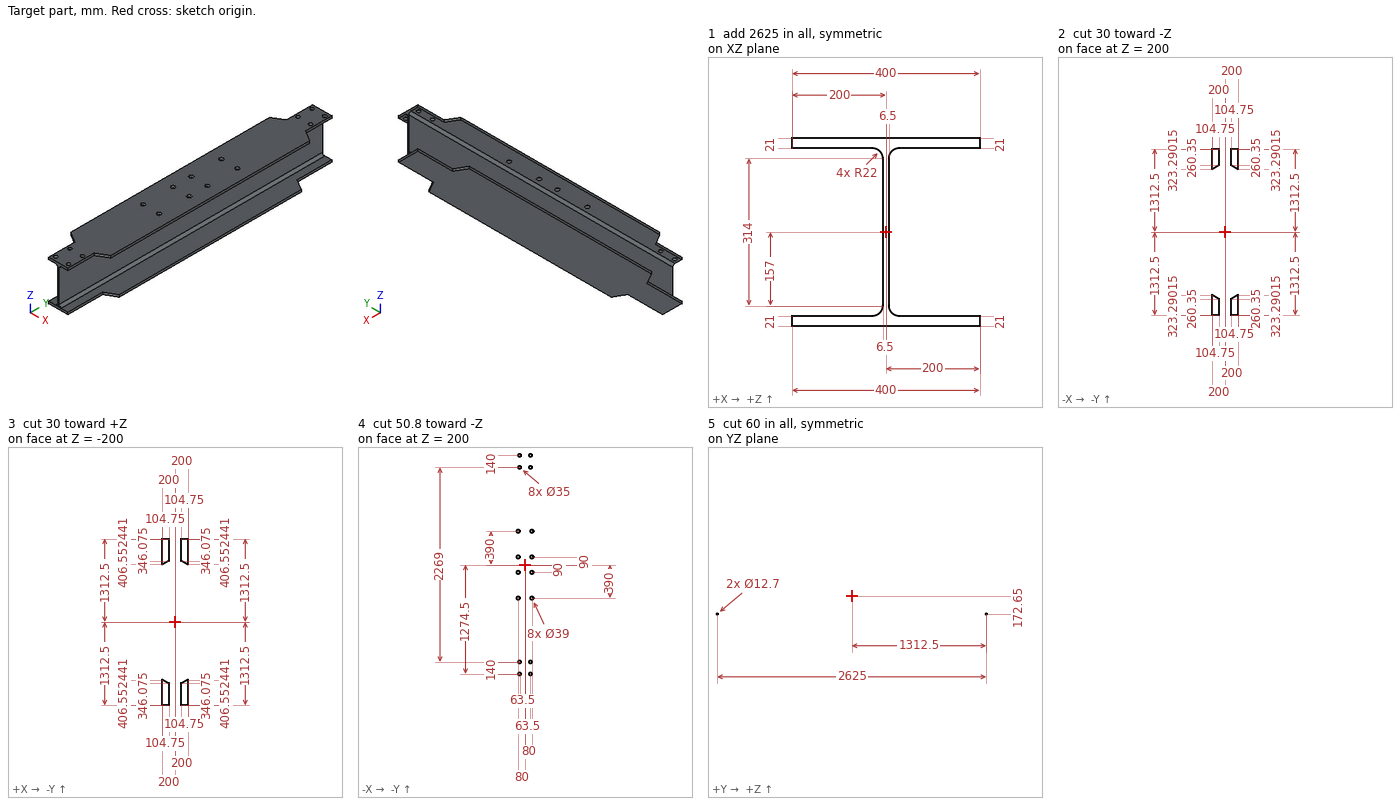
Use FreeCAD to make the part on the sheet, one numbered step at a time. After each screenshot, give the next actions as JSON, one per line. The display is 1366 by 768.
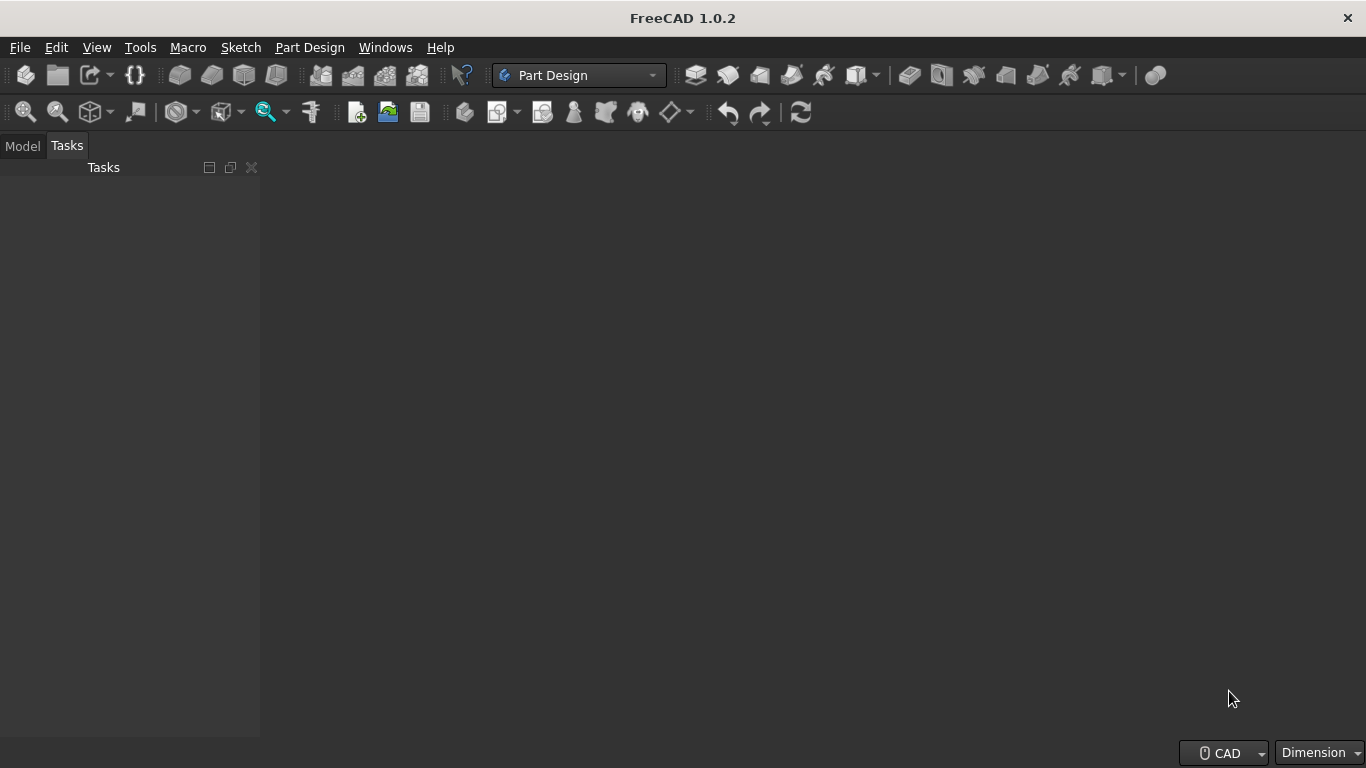
{"action": "left_click", "coordinate": [356, 112]}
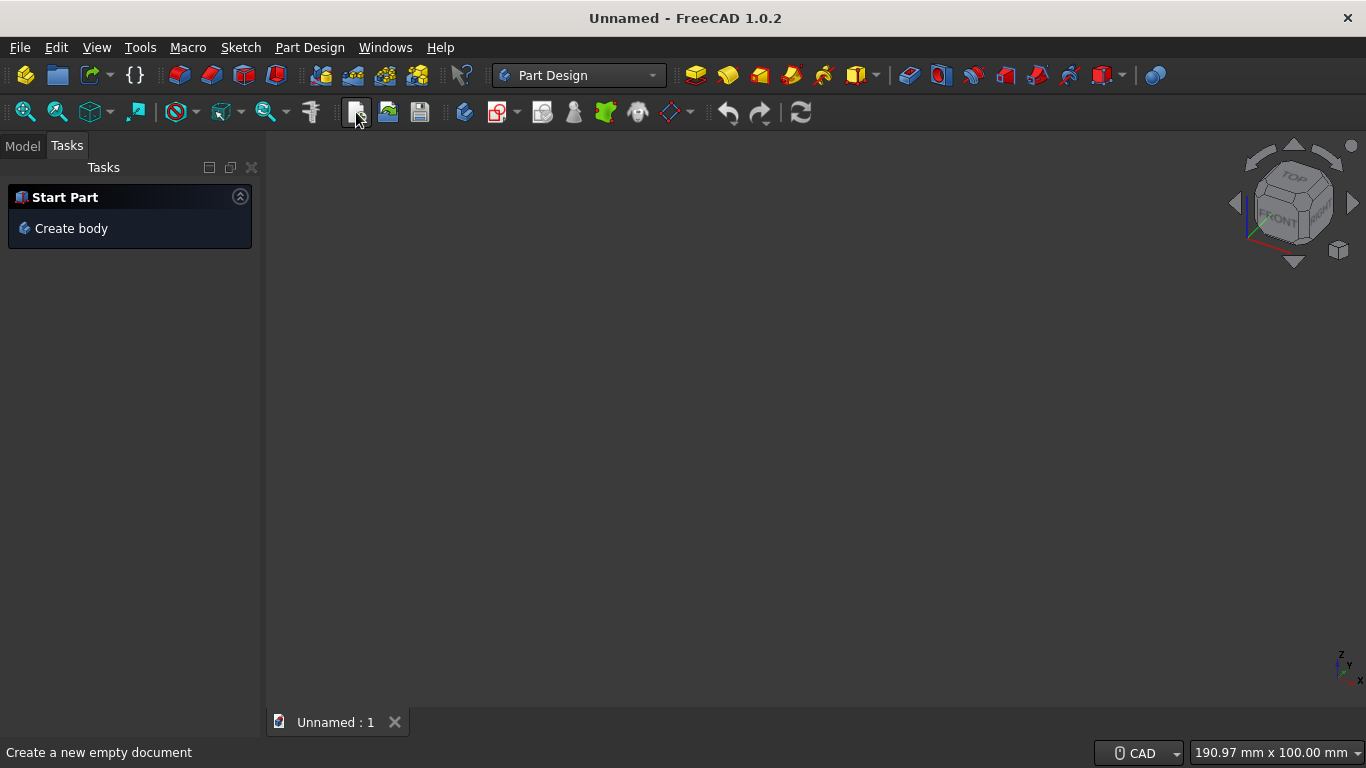
{"action": "left_click", "coordinate": [498, 112]}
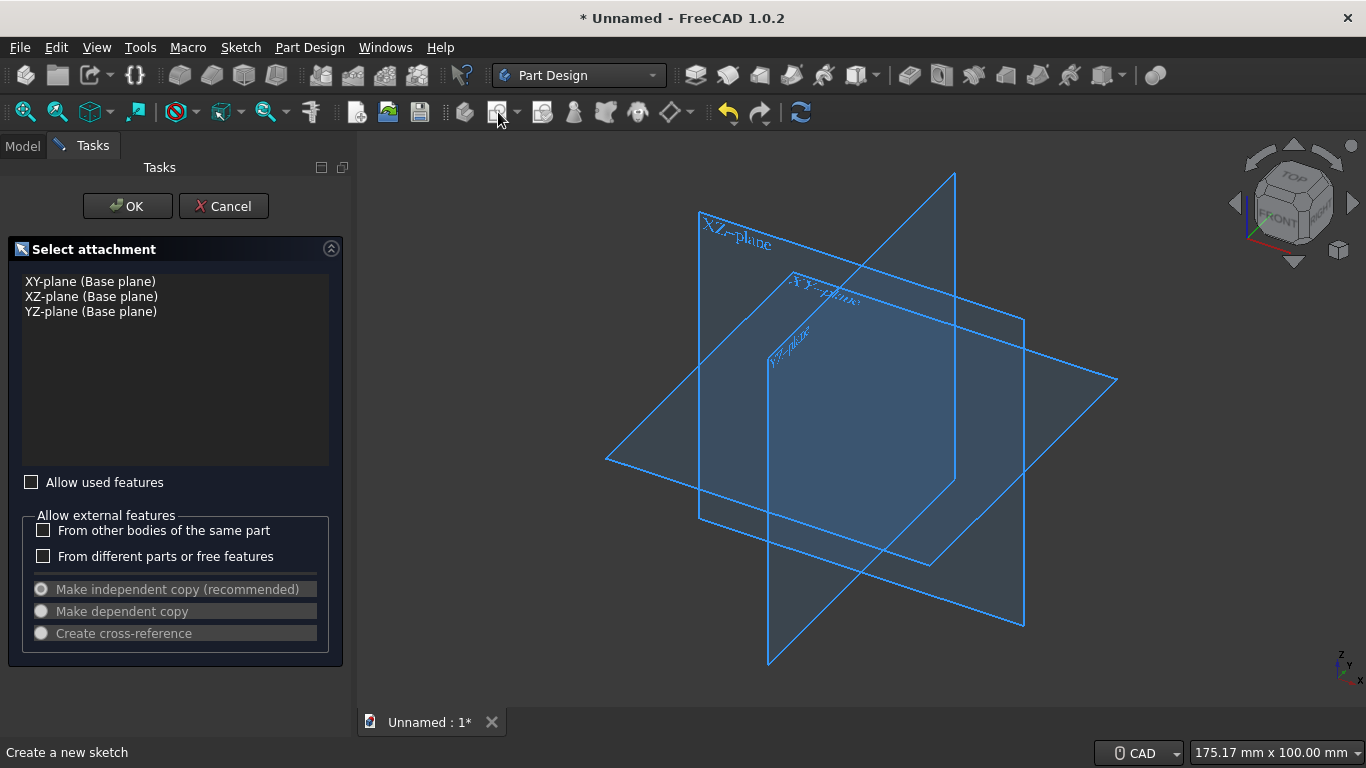
{"action": "left_click", "coordinate": [82, 296]}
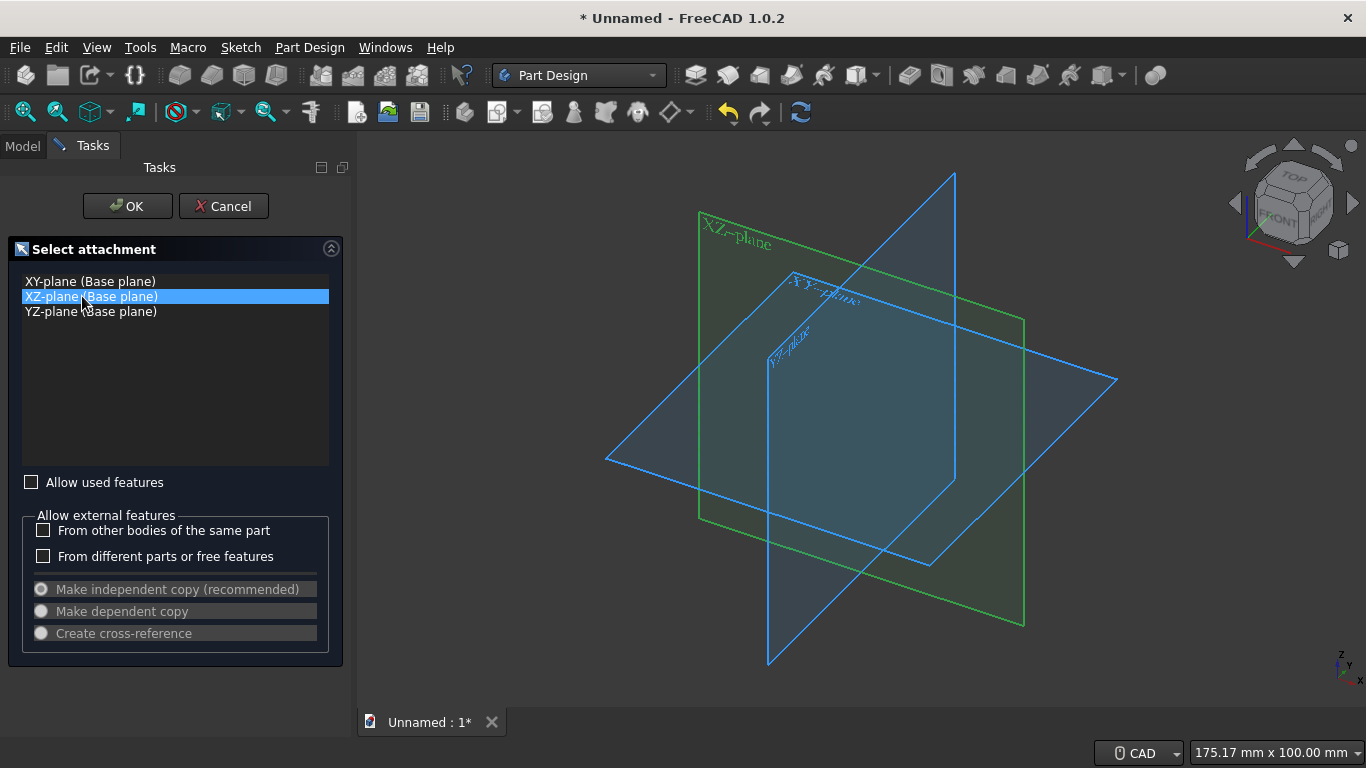
{"action": "left_click", "coordinate": [128, 206]}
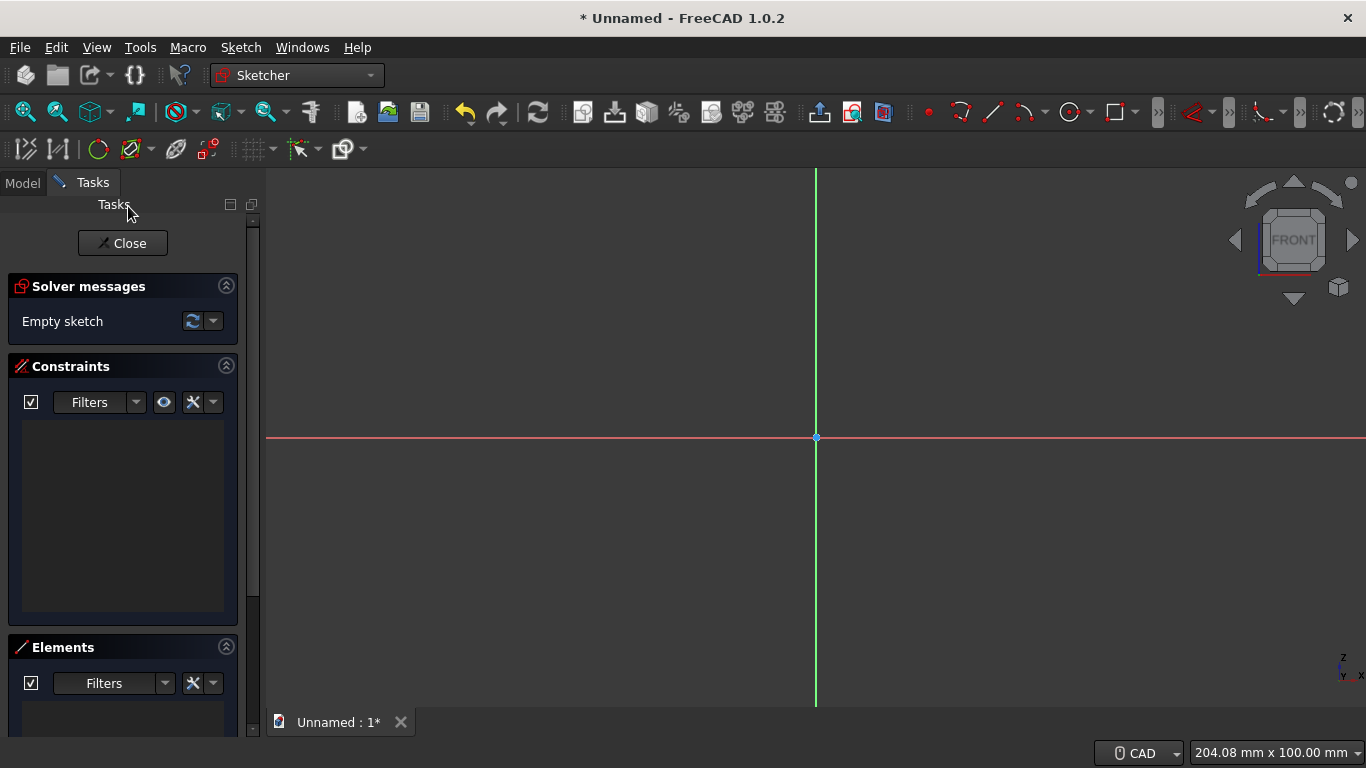
{"action": "scroll", "coordinate": [734, 438], "scroll_direction": "down", "scroll_amount": 9}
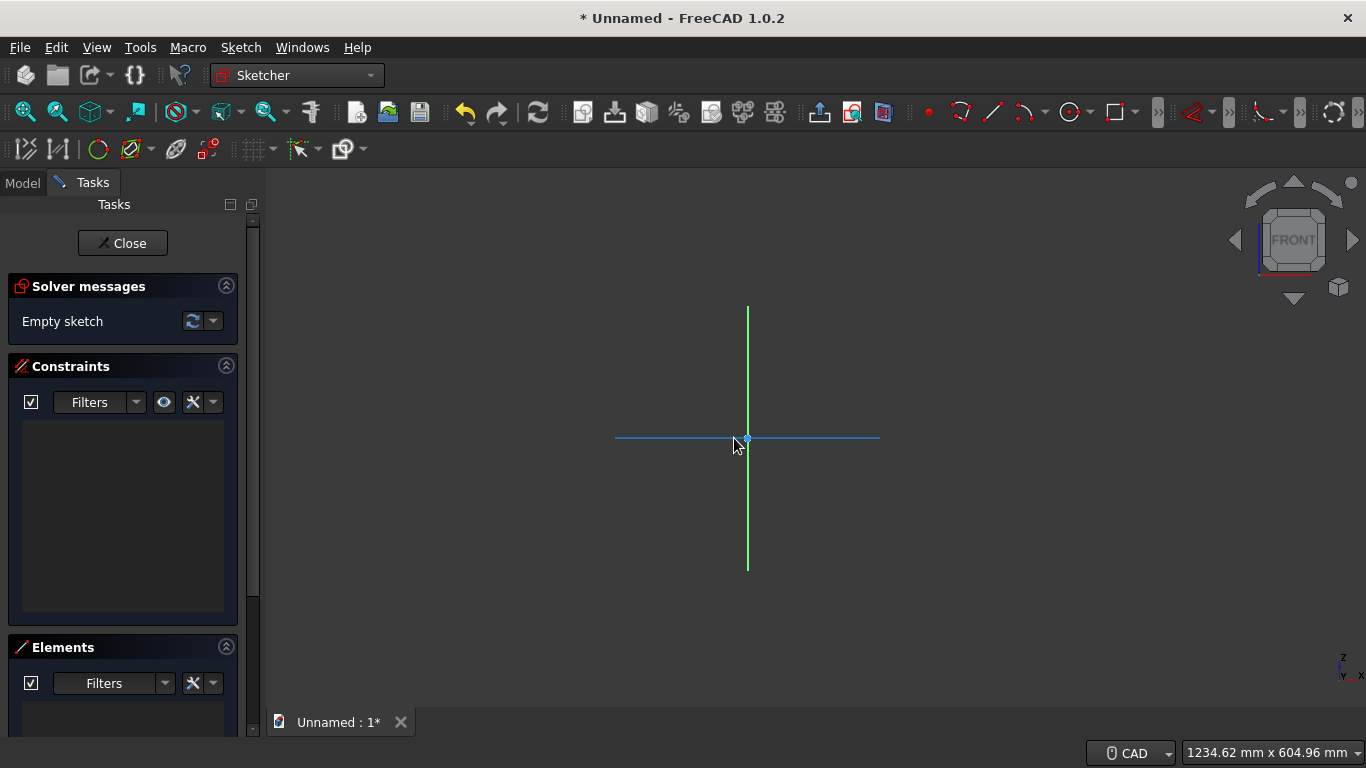
{"action": "left_click", "coordinate": [994, 112]}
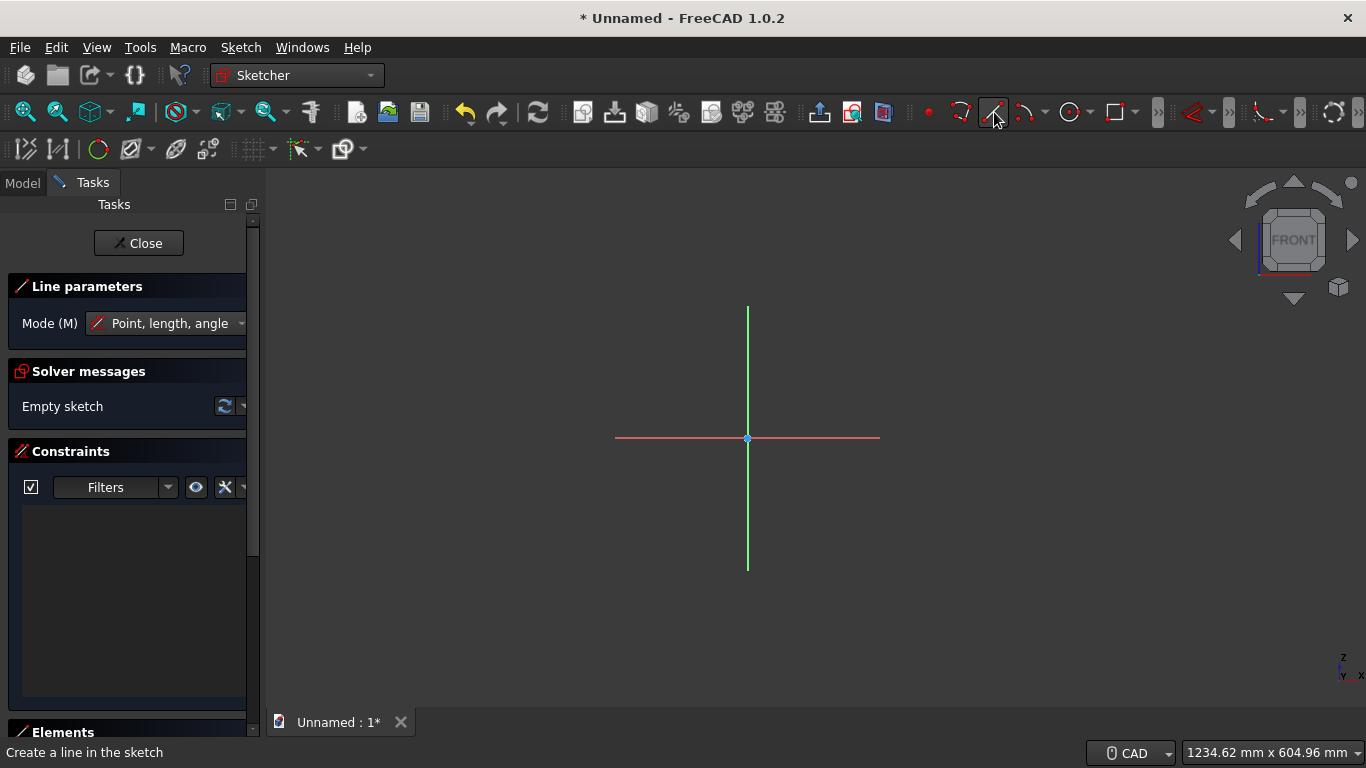
{"action": "scroll", "coordinate": [742, 578], "scroll_direction": "up", "scroll_amount": 6}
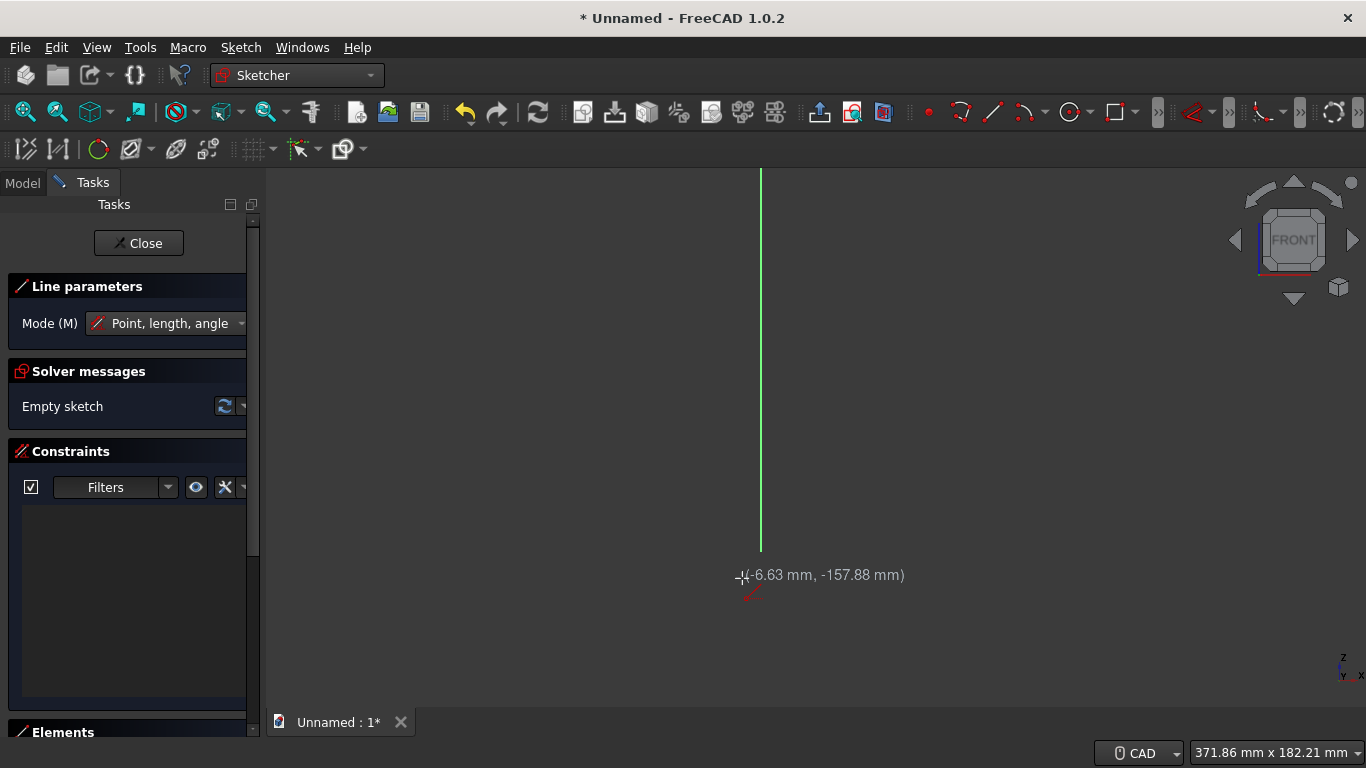
{"action": "left_click", "coordinate": [741, 577]}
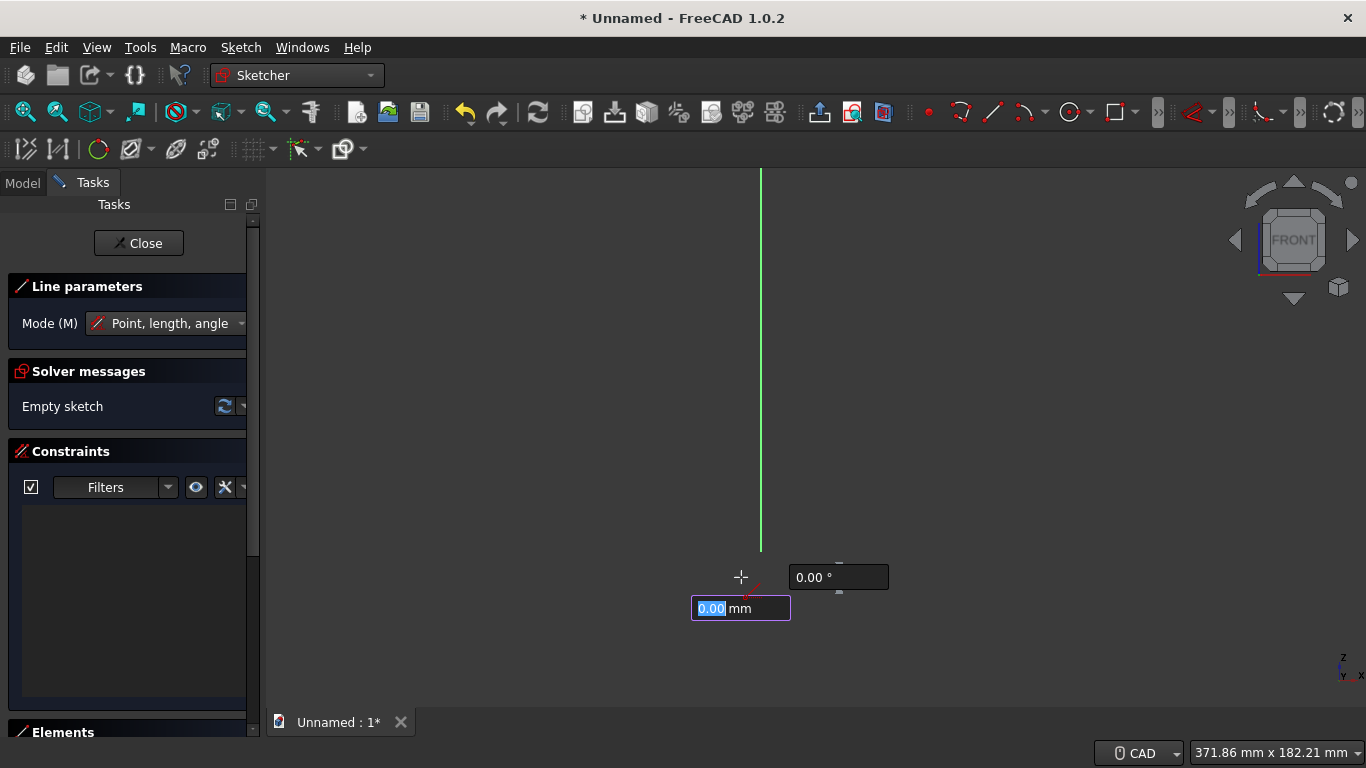
{"action": "scroll", "coordinate": [742, 578], "scroll_direction": "down", "scroll_amount": 6}